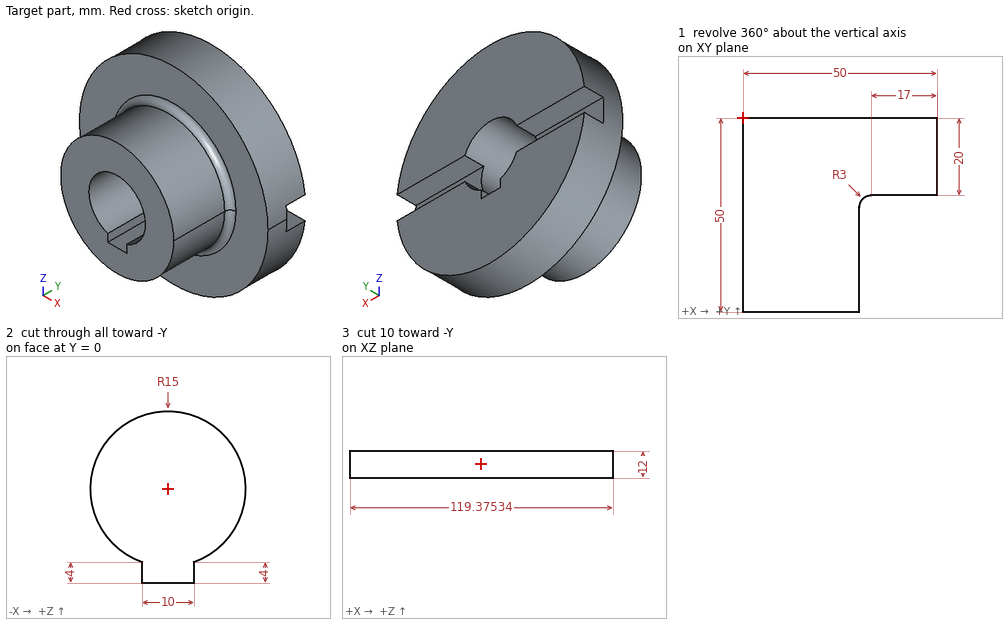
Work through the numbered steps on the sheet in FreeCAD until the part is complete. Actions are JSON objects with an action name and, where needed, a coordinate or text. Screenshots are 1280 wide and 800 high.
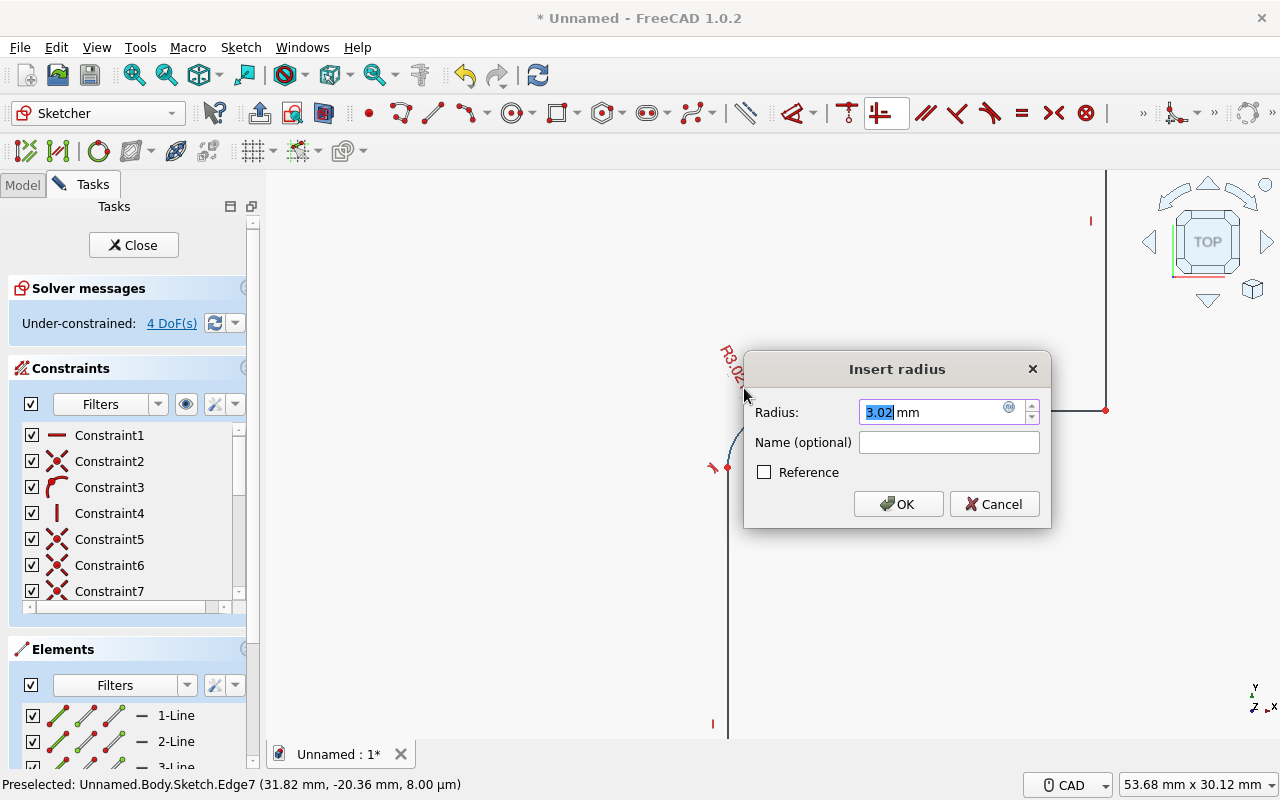
{"action": "type", "text": "3"}
{"action": "key", "text": "Return"}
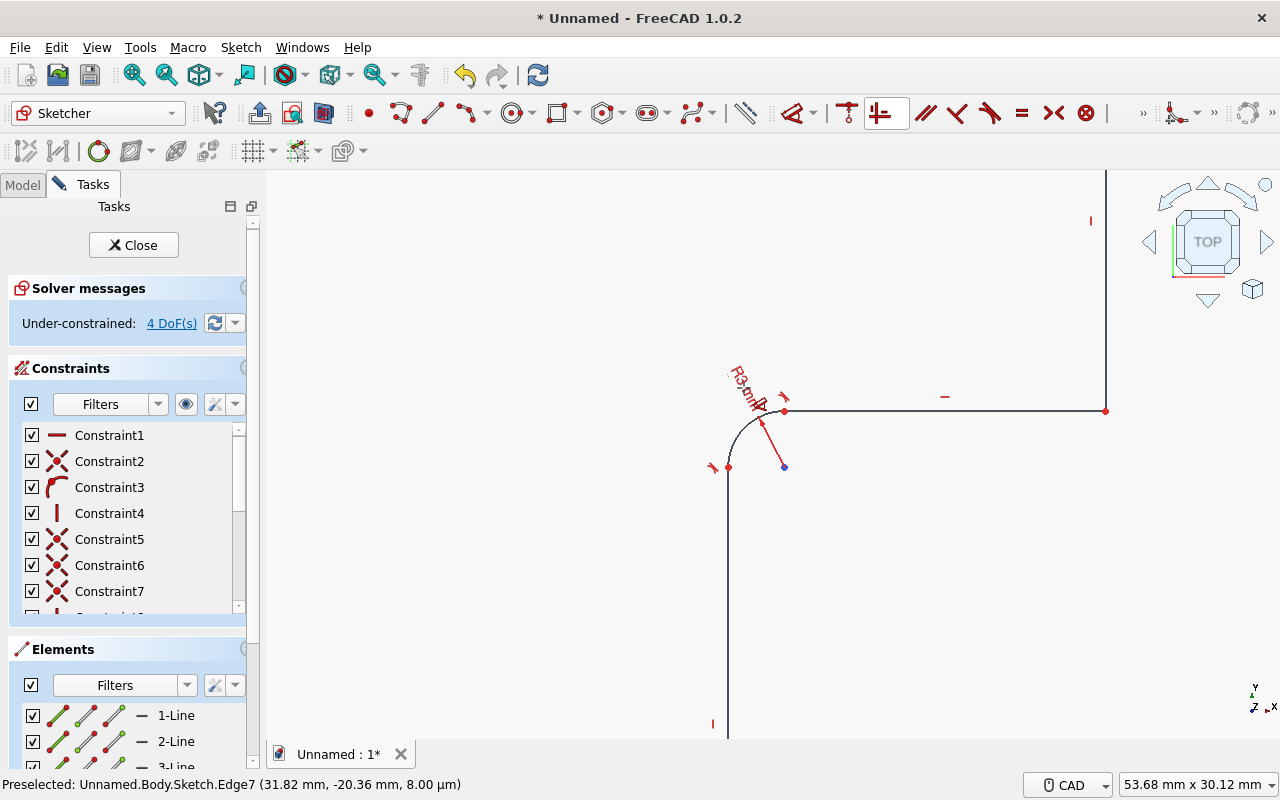
{"action": "left_click", "coordinate": [881, 411]}
{"action": "left_click", "coordinate": [945, 377]}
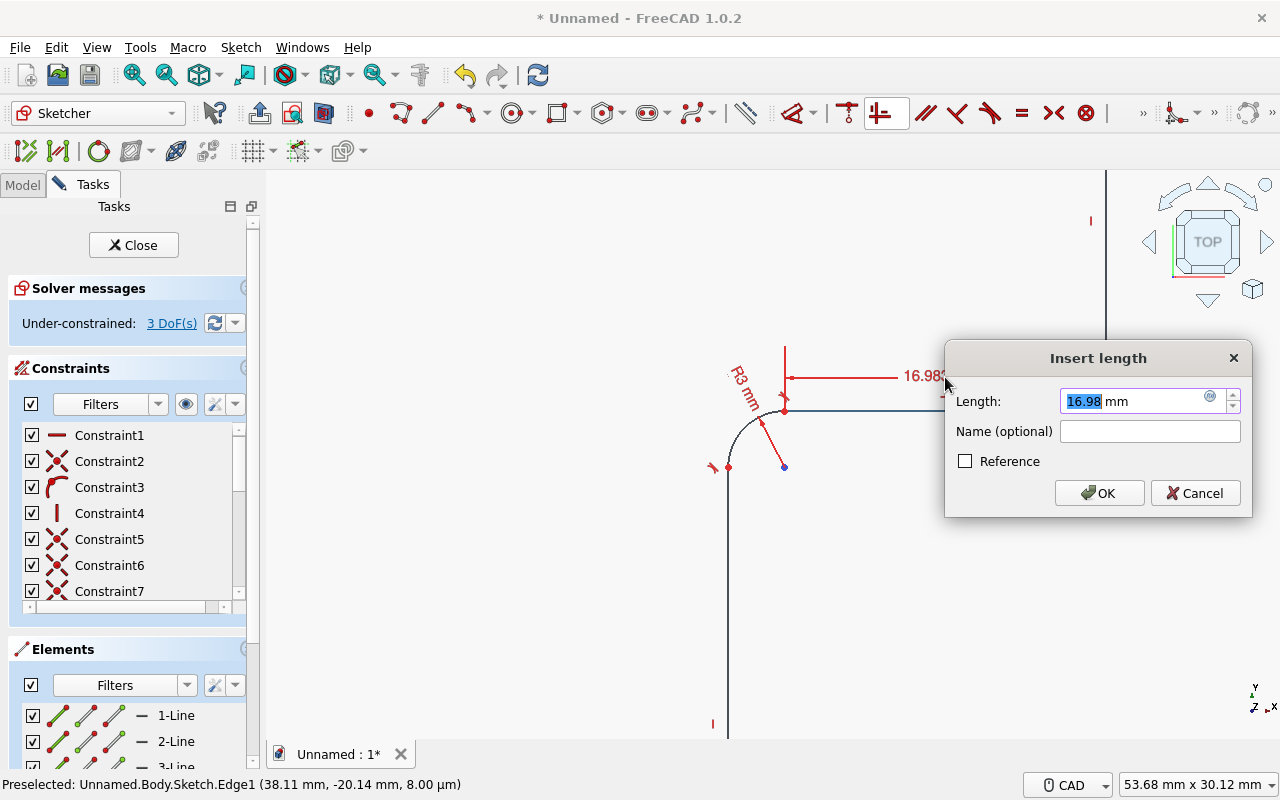
{"action": "type", "text": "17"}
{"action": "key", "text": "Return"}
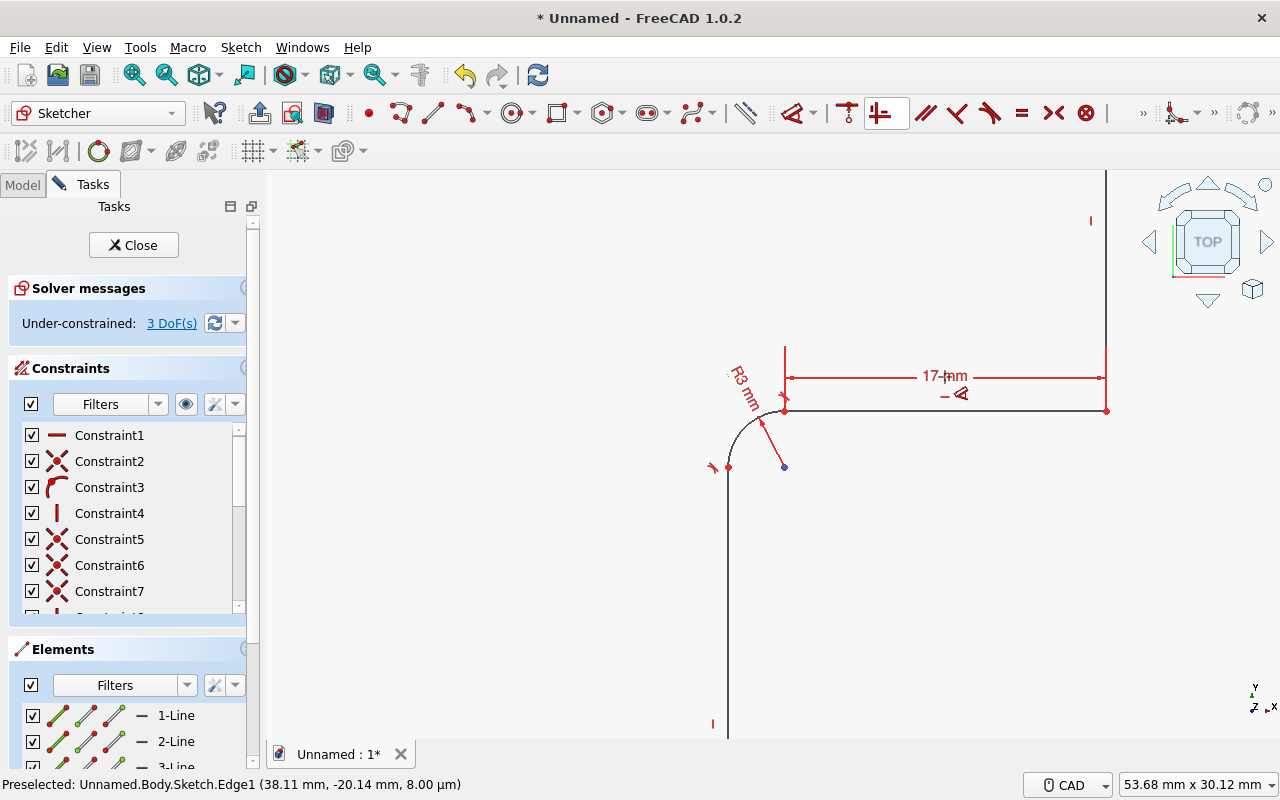
{"action": "left_click", "coordinate": [1106, 297]}
{"action": "left_click", "coordinate": [1072, 305]}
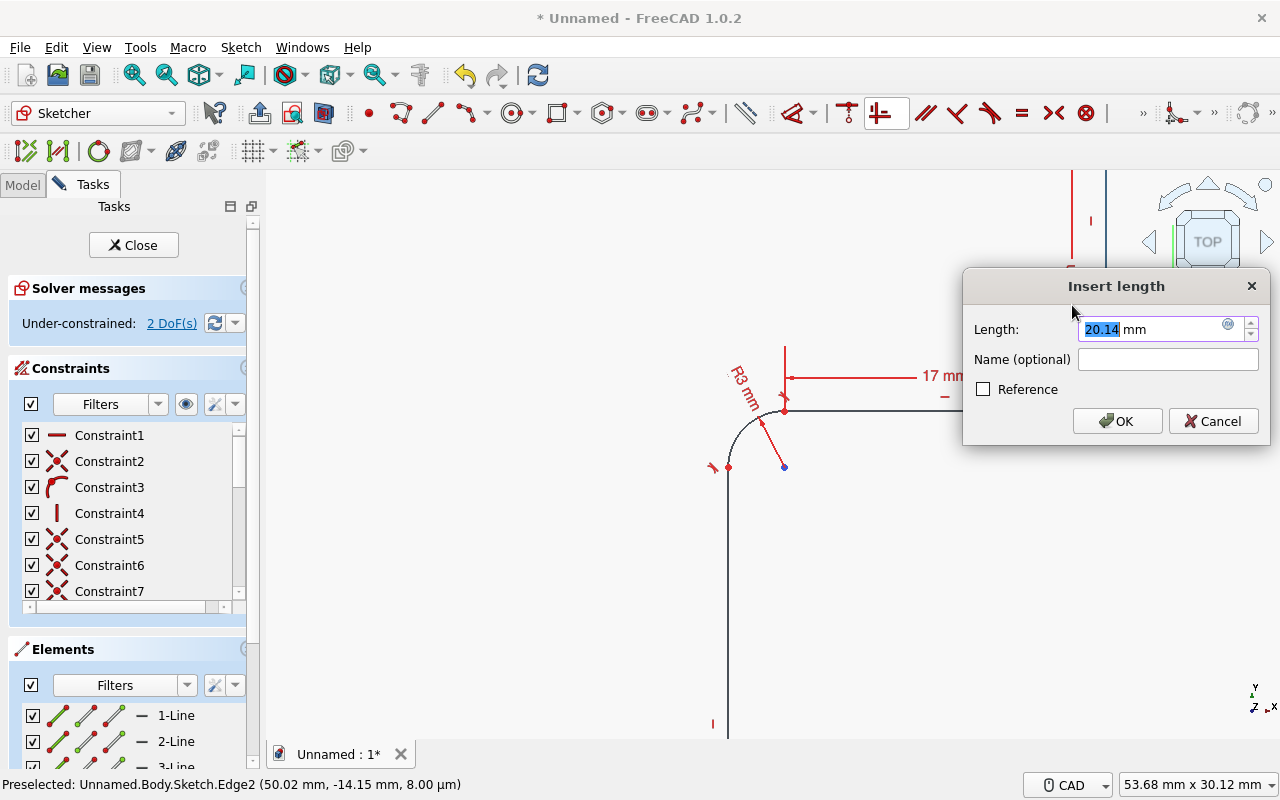
{"action": "type", "text": "20"}
{"action": "key", "text": "Return"}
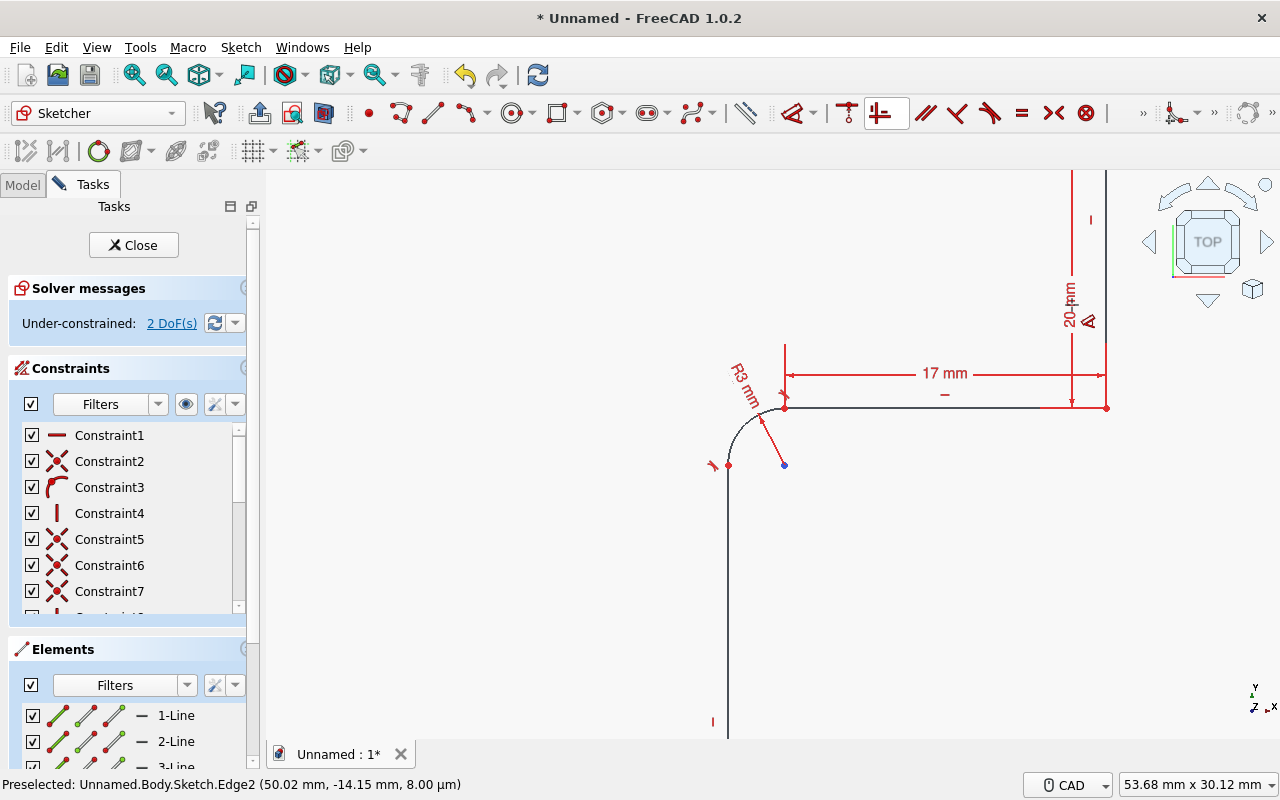
{"action": "scroll", "coordinate": [746, 426], "scroll_direction": "down", "scroll_amount": 5}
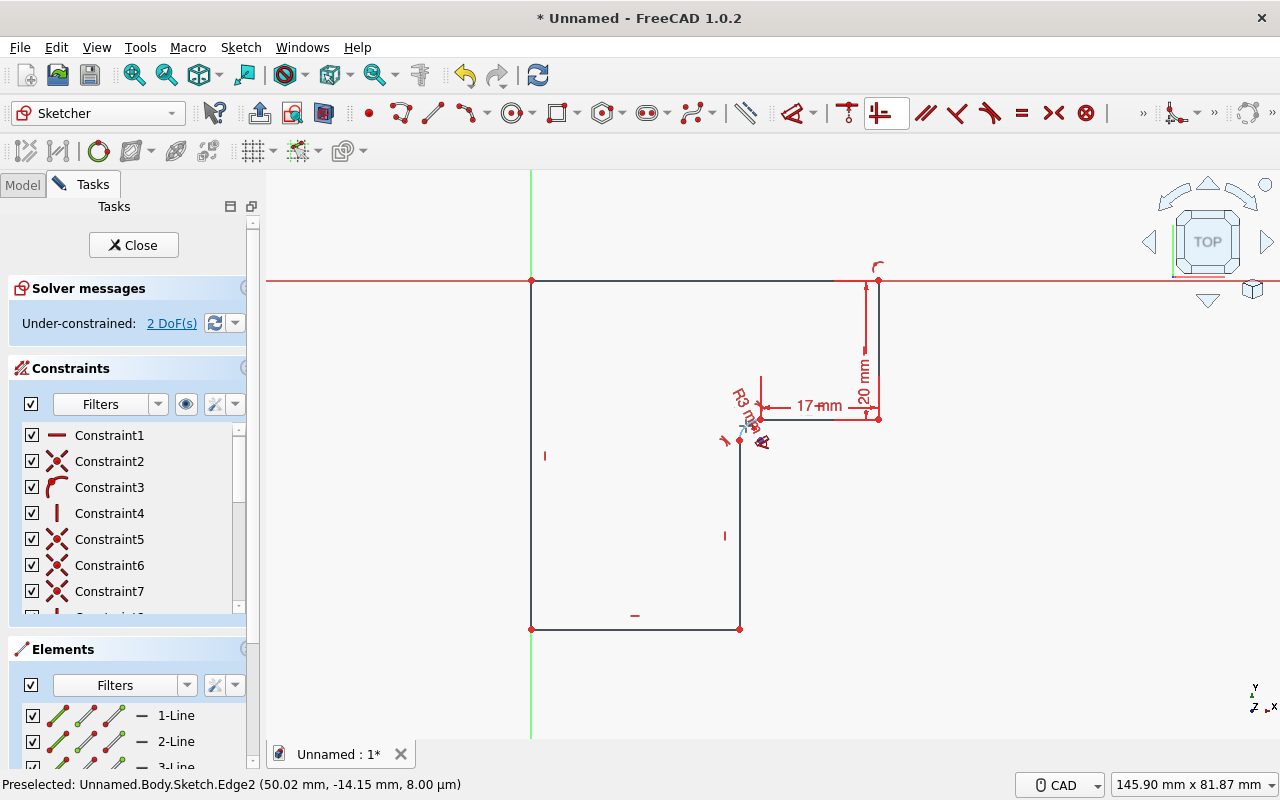
{"action": "left_click", "coordinate": [774, 281]}
{"action": "left_click", "coordinate": [705, 247]}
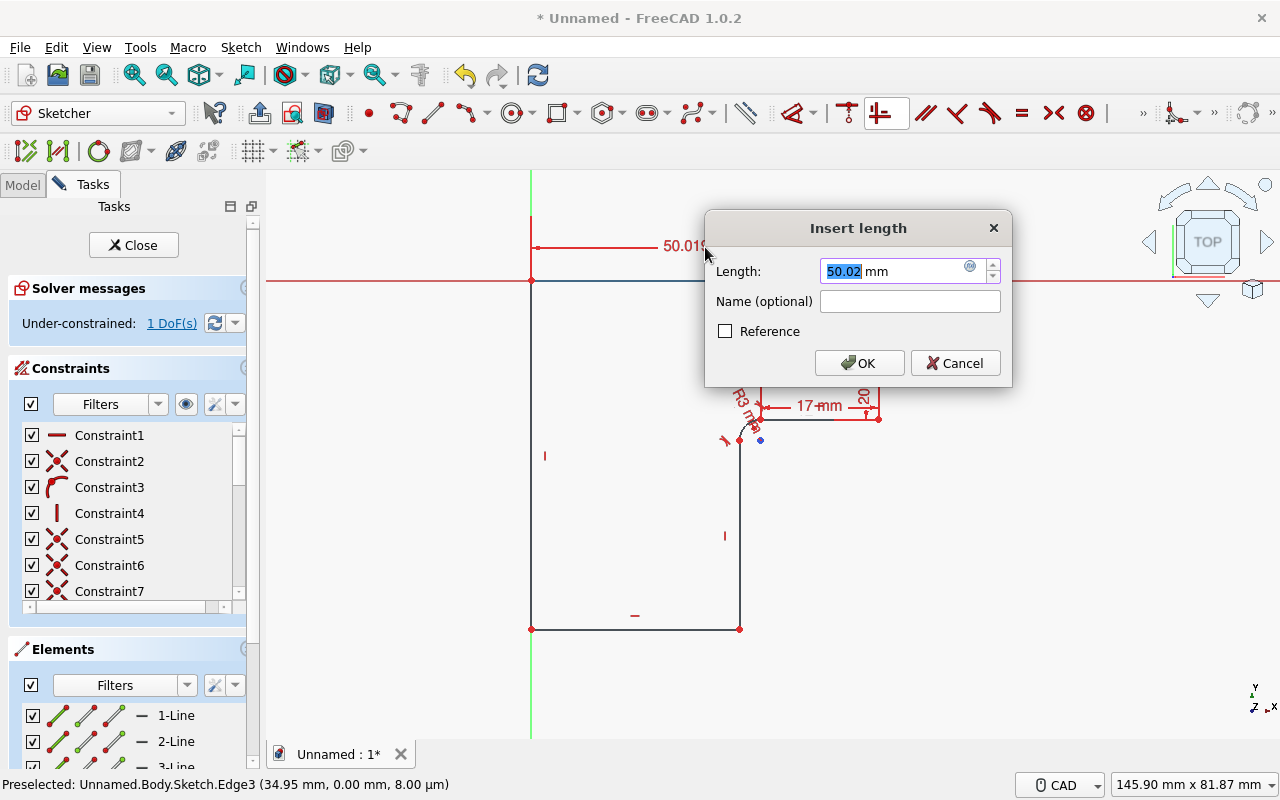
{"action": "type", "text": "50"}
{"action": "key", "text": "Return"}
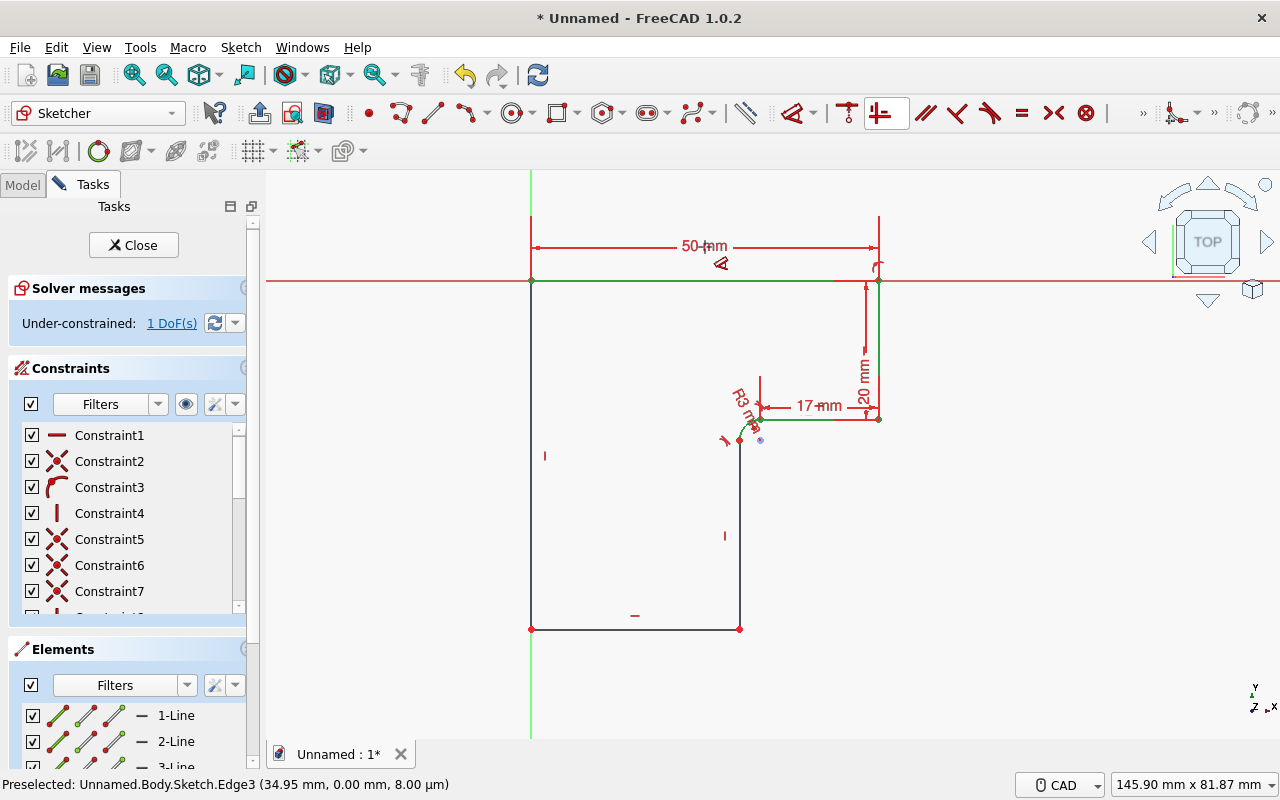
{"action": "left_click", "coordinate": [531, 385]}
{"action": "left_click", "coordinate": [497, 455]}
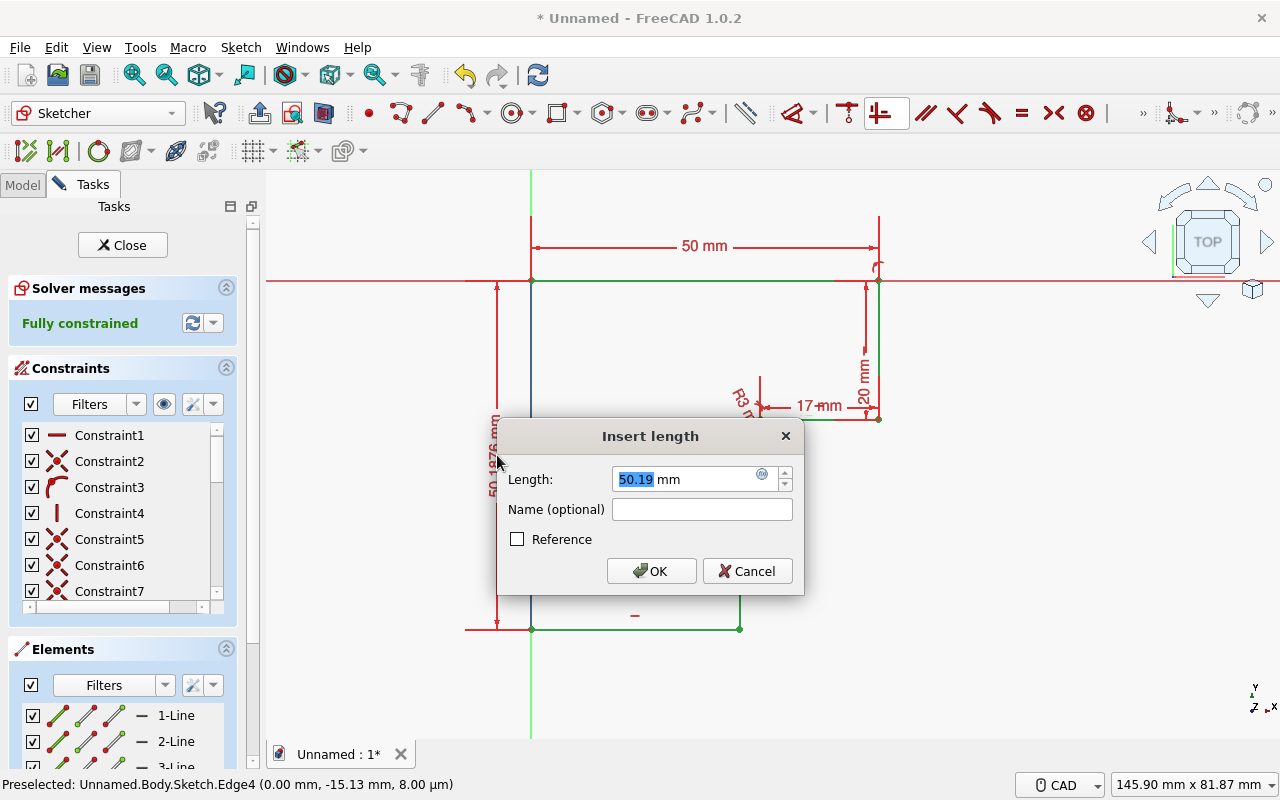
{"action": "type", "text": "50"}
{"action": "key", "text": "Return"}
{"action": "key", "text": "Escape"}